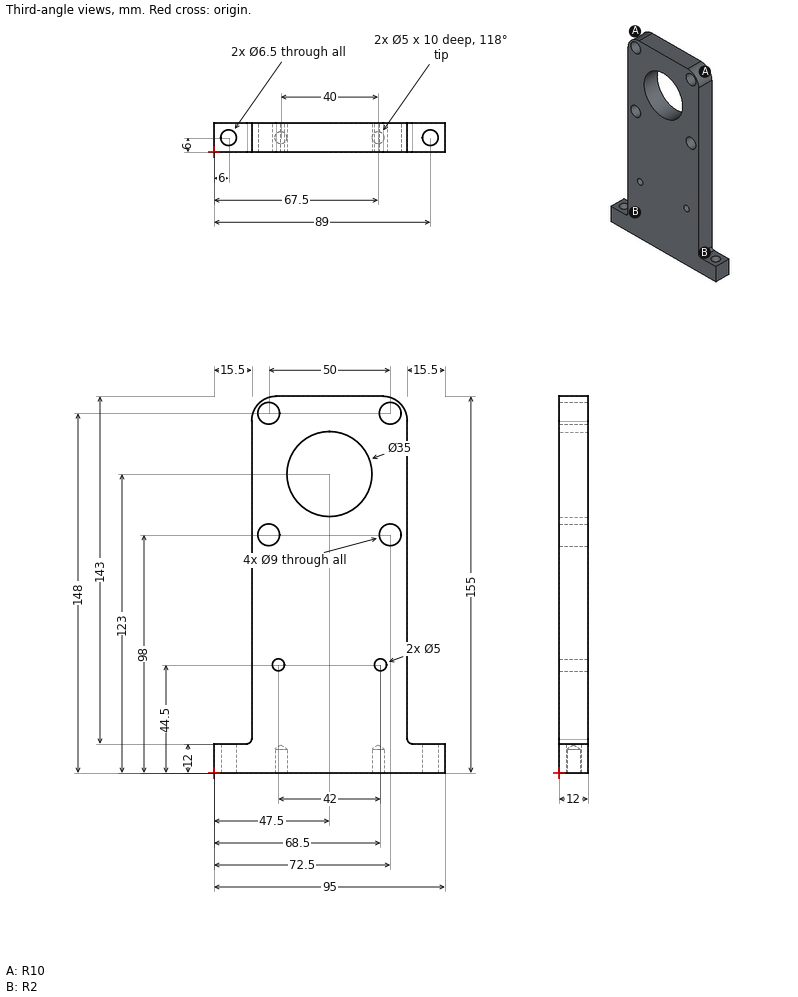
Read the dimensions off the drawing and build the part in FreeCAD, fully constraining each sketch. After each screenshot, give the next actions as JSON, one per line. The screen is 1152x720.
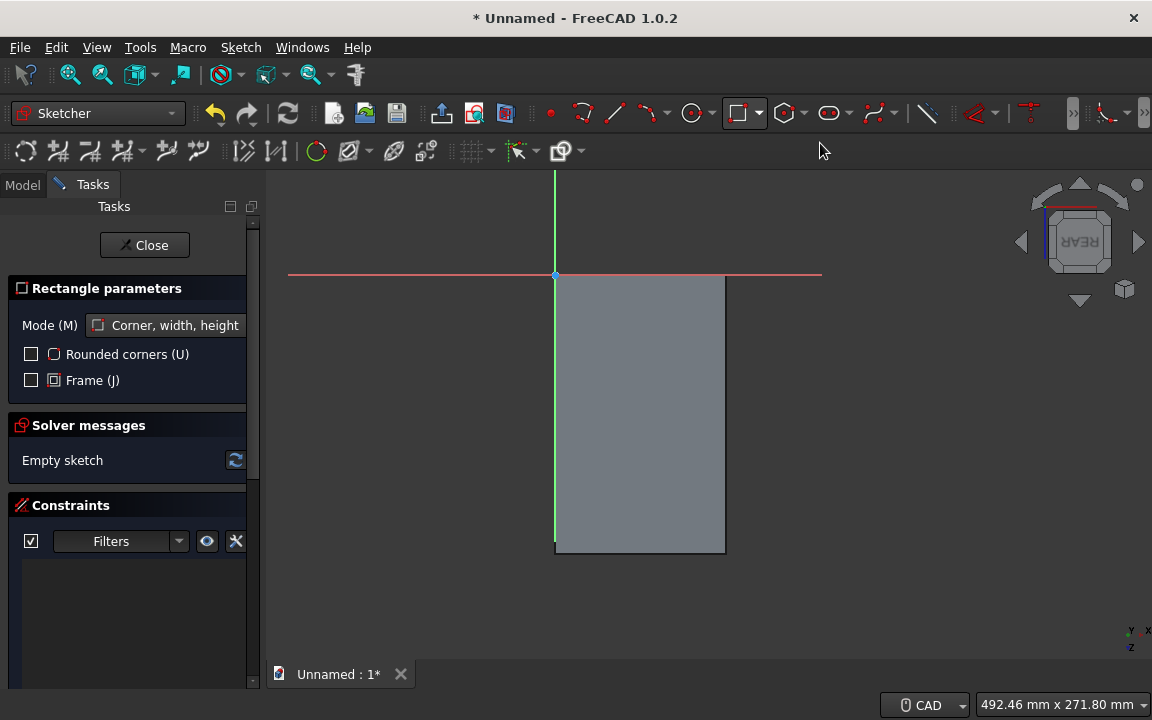
{"action": "left_click", "coordinate": [555, 297]}
{"action": "left_click", "coordinate": [583, 554]}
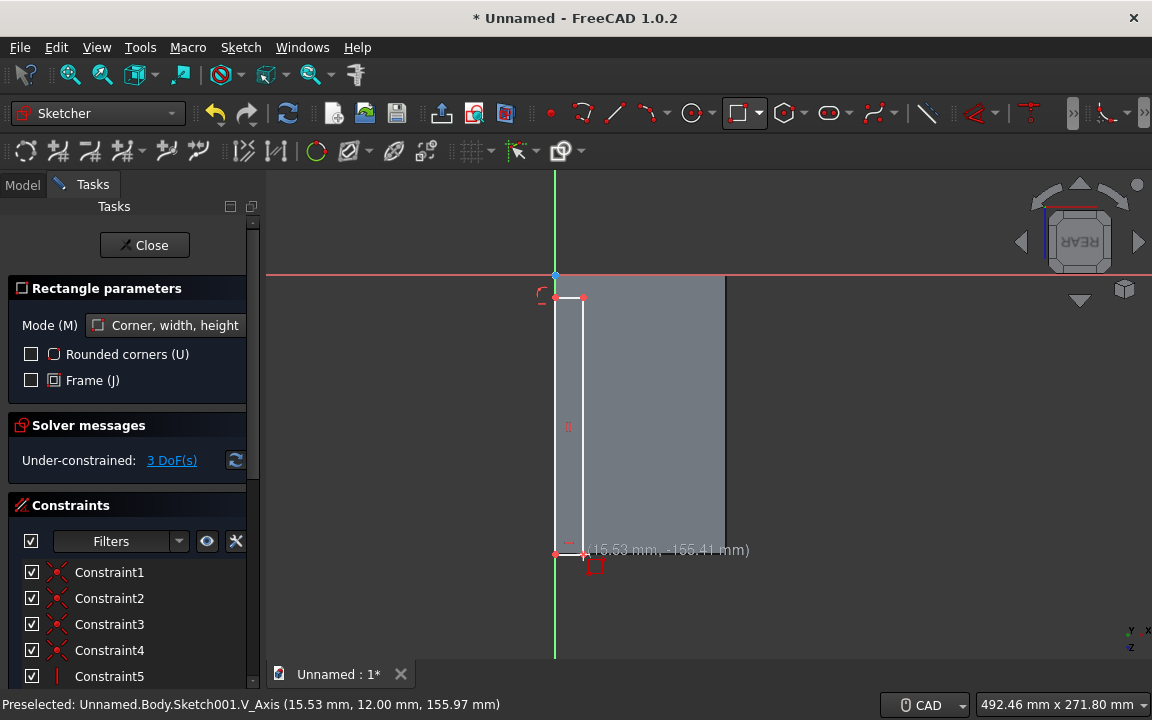
{"action": "left_click", "coordinate": [698, 297]}
{"action": "left_click", "coordinate": [726, 554]}
{"action": "key", "text": "Escape"}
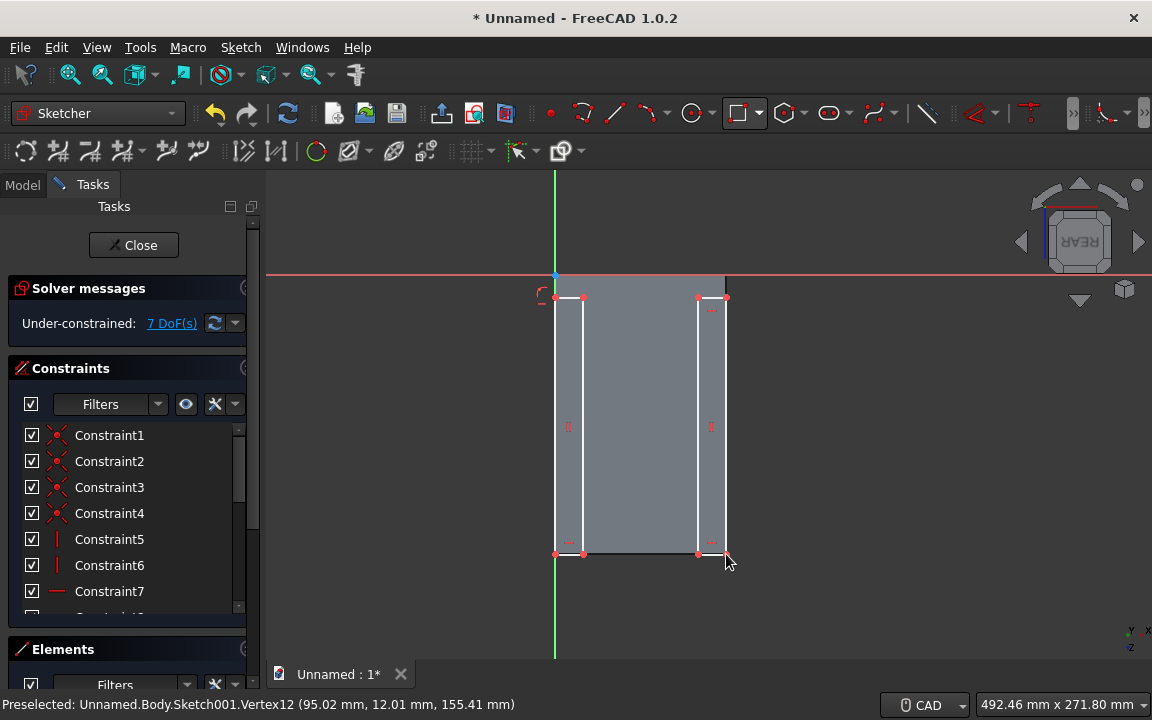
{"action": "left_click", "coordinate": [974, 114]}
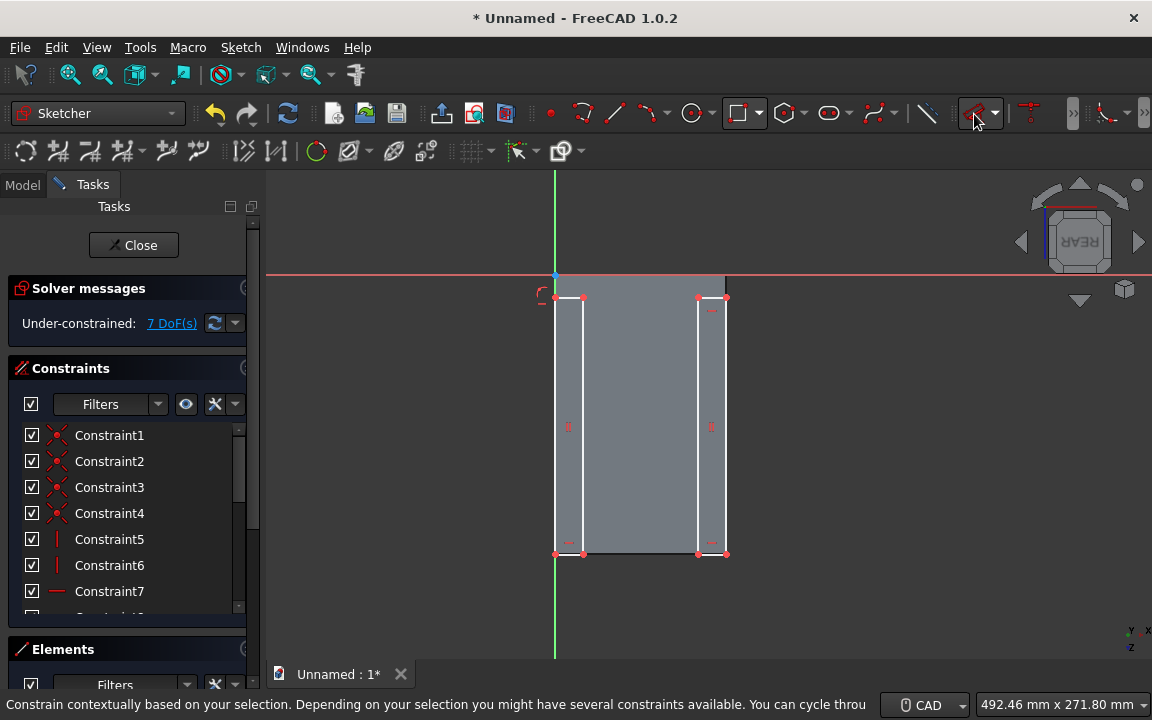
{"action": "left_click", "coordinate": [555, 375]}
{"action": "left_click", "coordinate": [521, 427]}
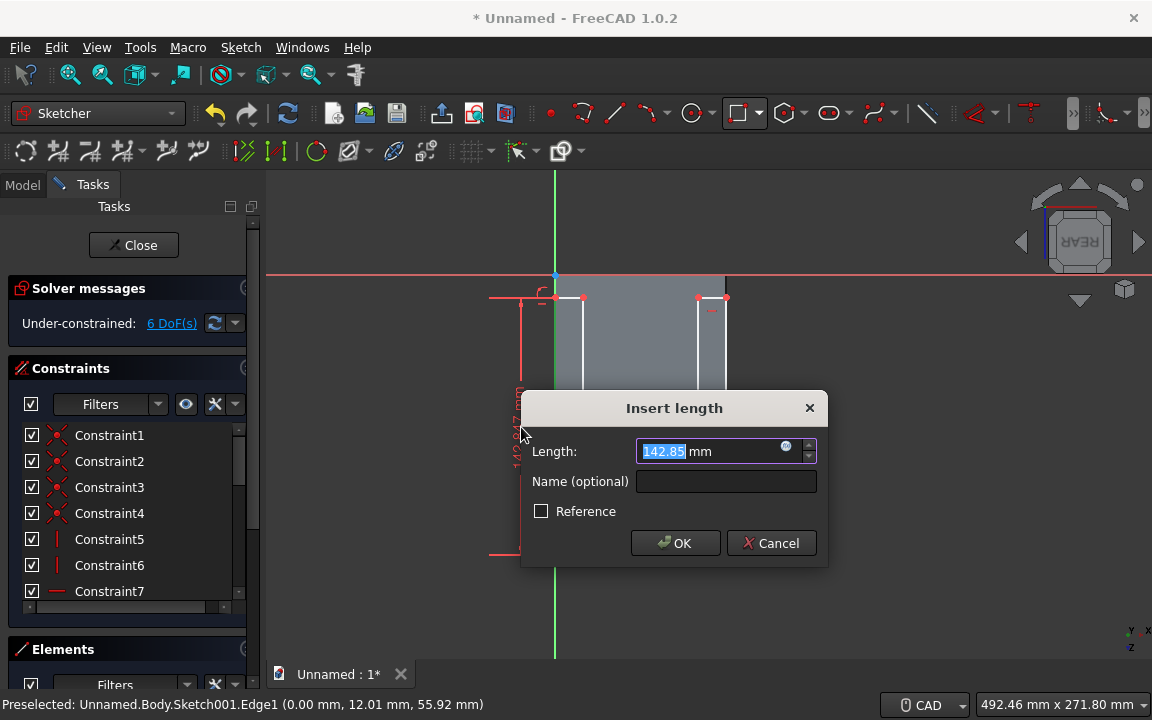
{"action": "type", "text": "143"}
{"action": "key", "text": "Return"}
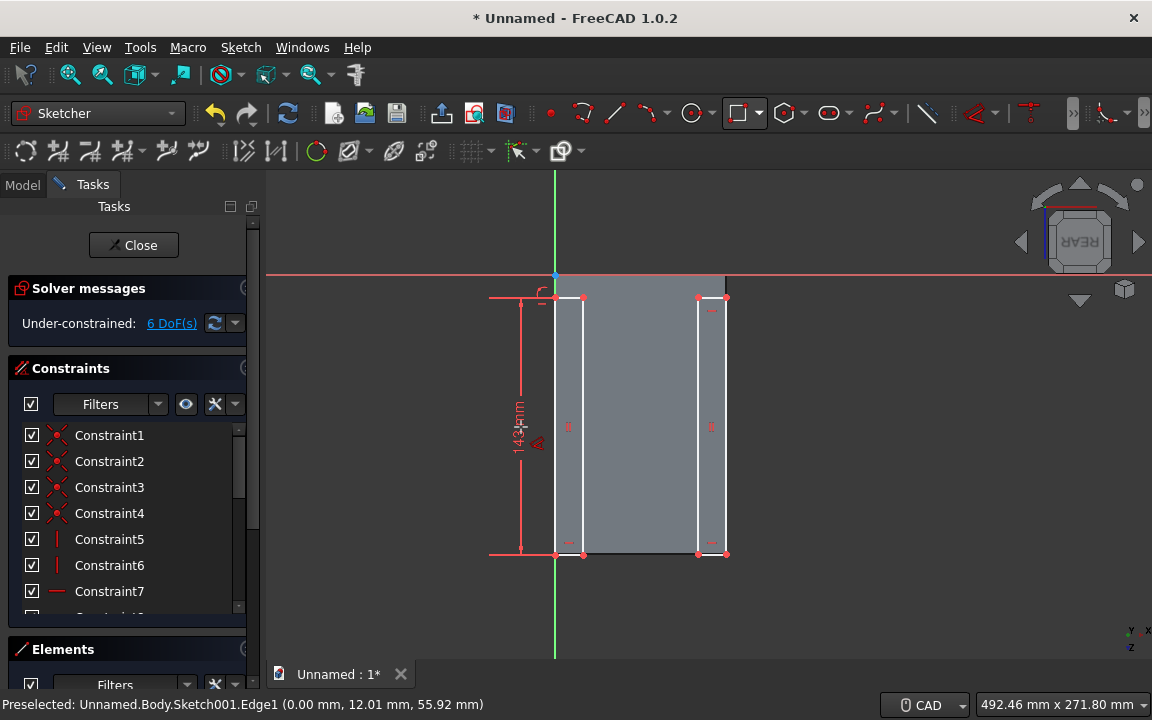
{"action": "left_click", "coordinate": [698, 375]}
{"action": "left_click", "coordinate": [664, 427]}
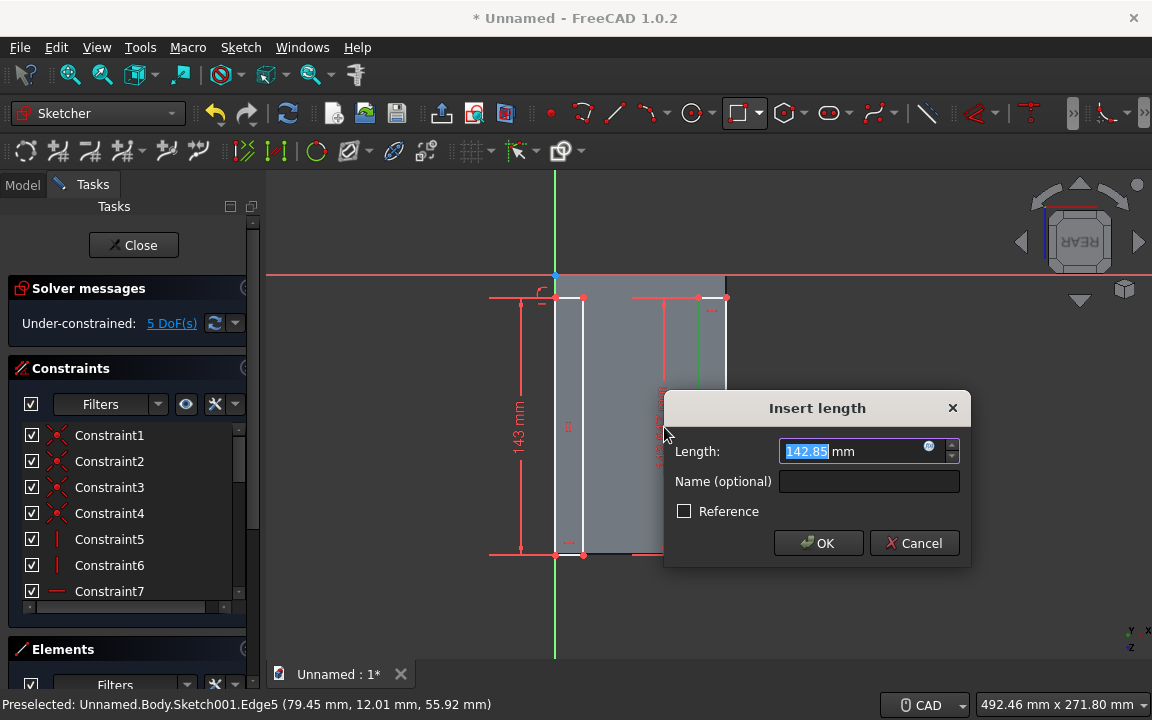
{"action": "type", "text": "143"}
{"action": "key", "text": "Return"}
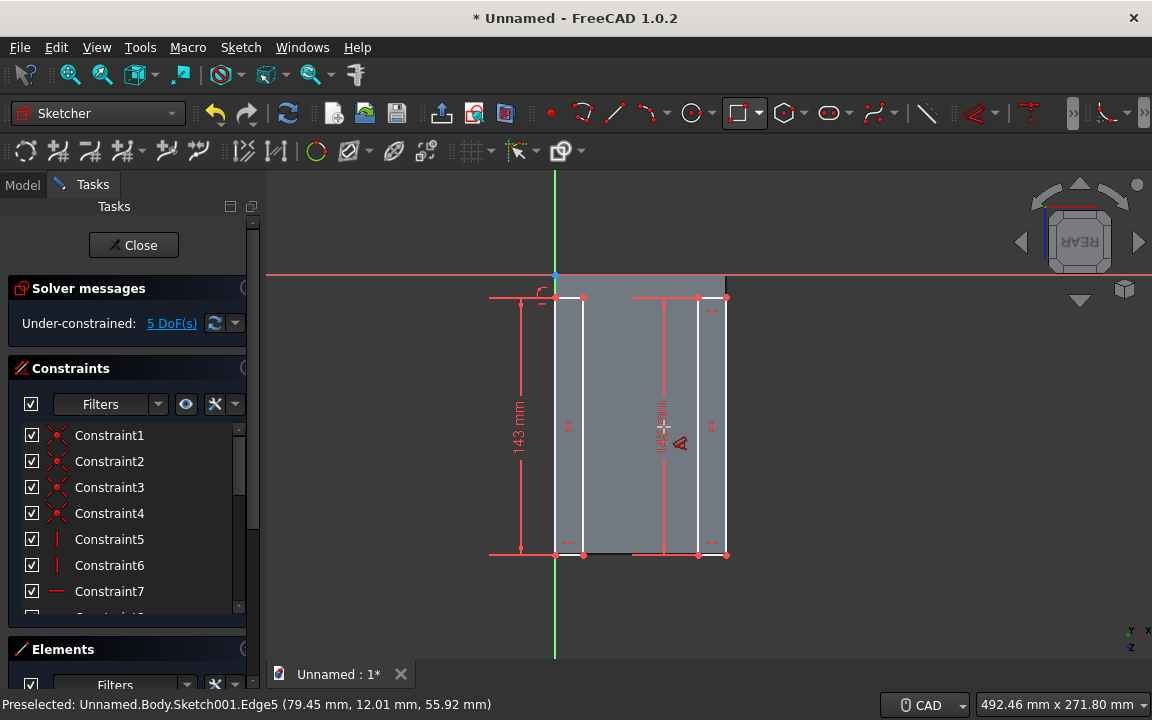
{"action": "scroll", "coordinate": [555, 298], "scroll_direction": "up", "scroll_amount": 4}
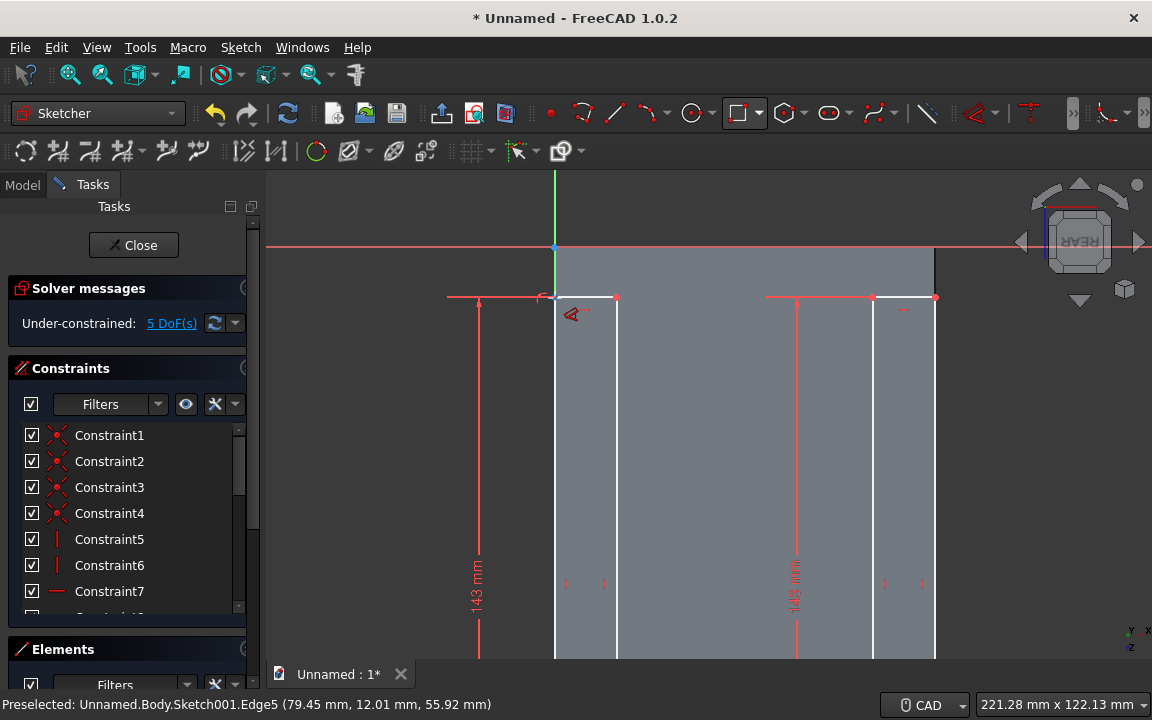
{"action": "left_click", "coordinate": [555, 297]}
{"action": "left_click", "coordinate": [521, 272]}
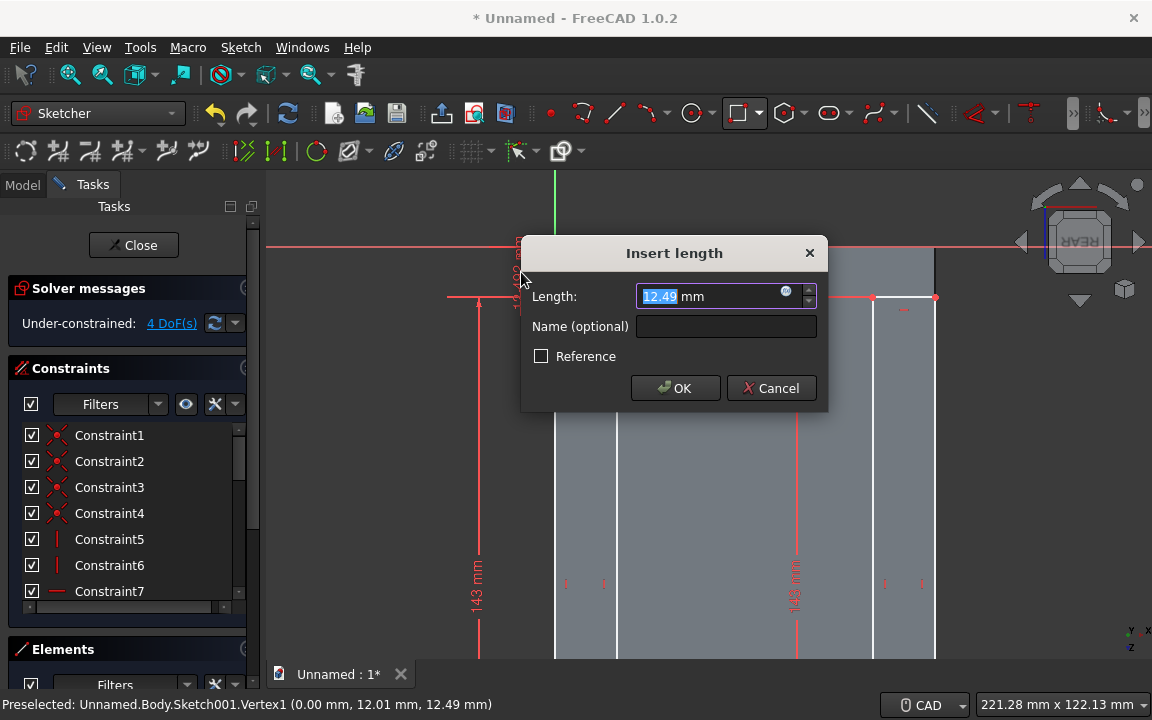
{"action": "type", "text": "12"}
{"action": "key", "text": "Return"}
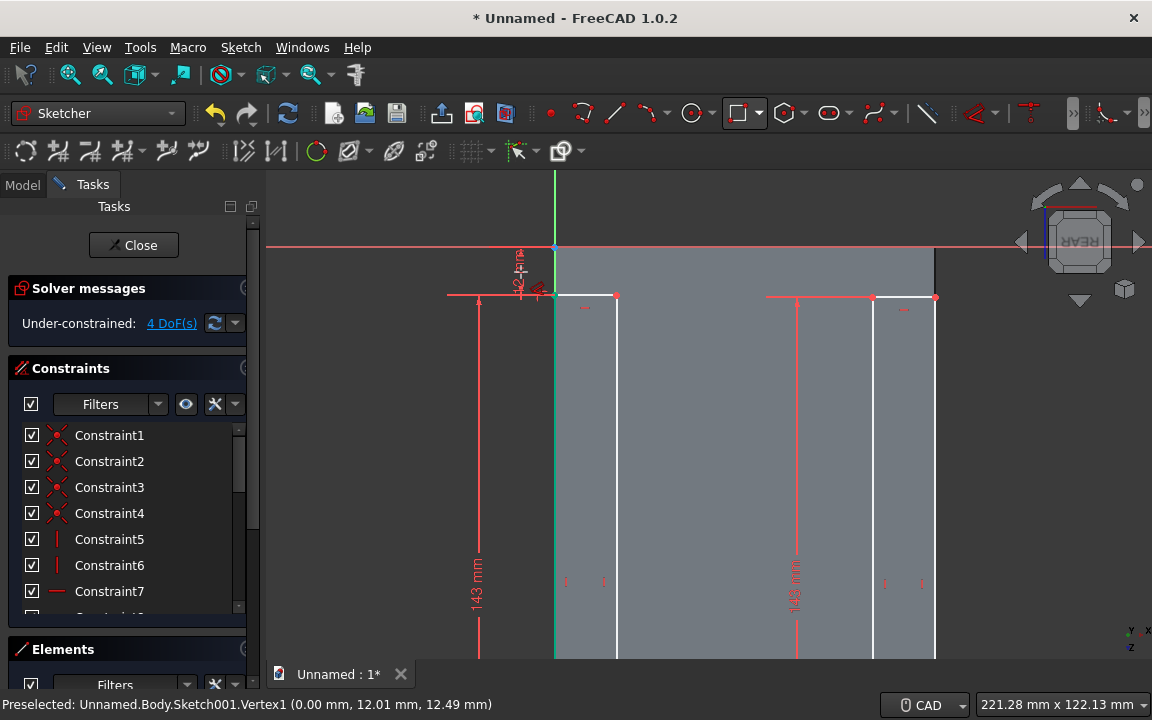
{"action": "left_click", "coordinate": [873, 297]}
{"action": "left_click", "coordinate": [907, 272]}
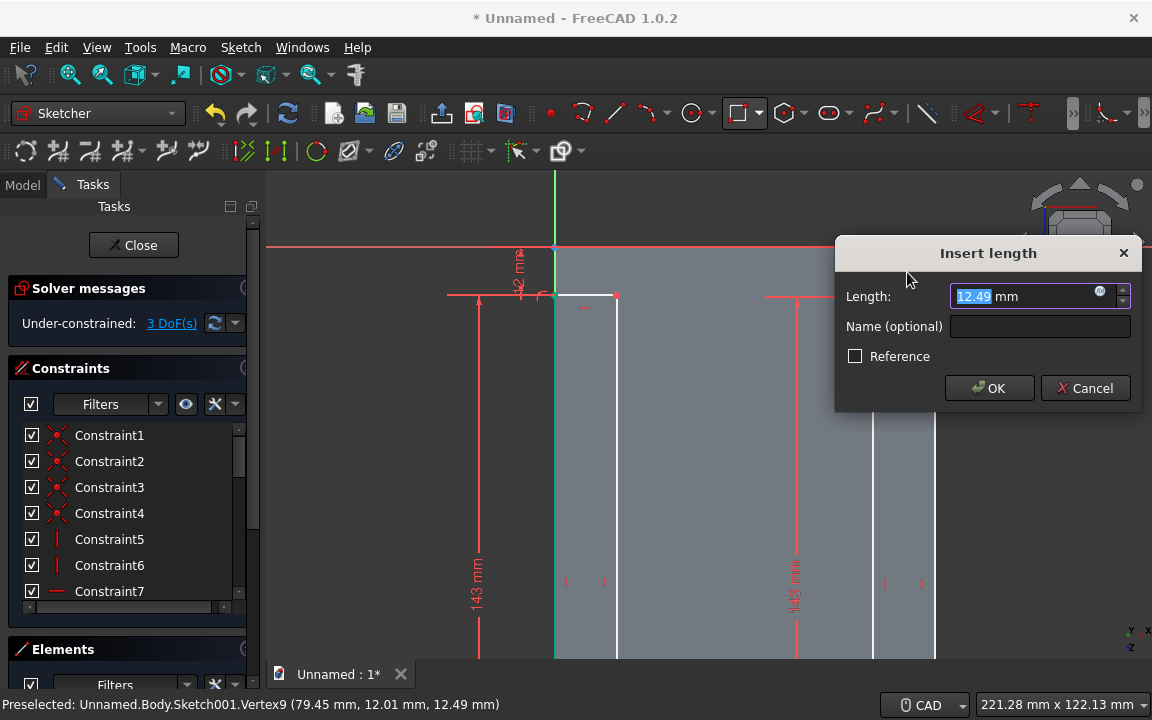
{"action": "type", "text": "12"}
{"action": "key", "text": "Return"}